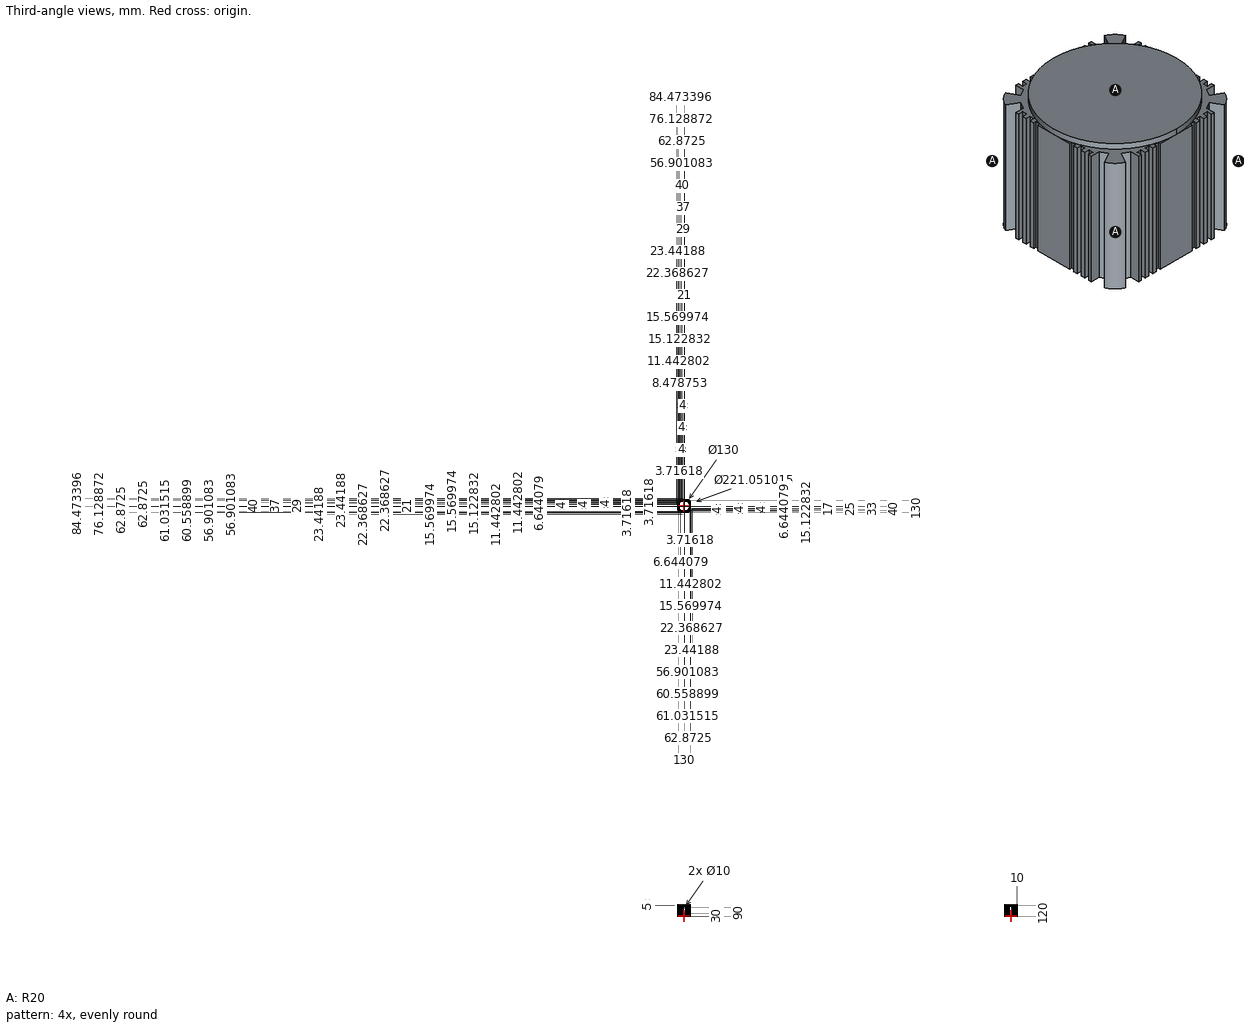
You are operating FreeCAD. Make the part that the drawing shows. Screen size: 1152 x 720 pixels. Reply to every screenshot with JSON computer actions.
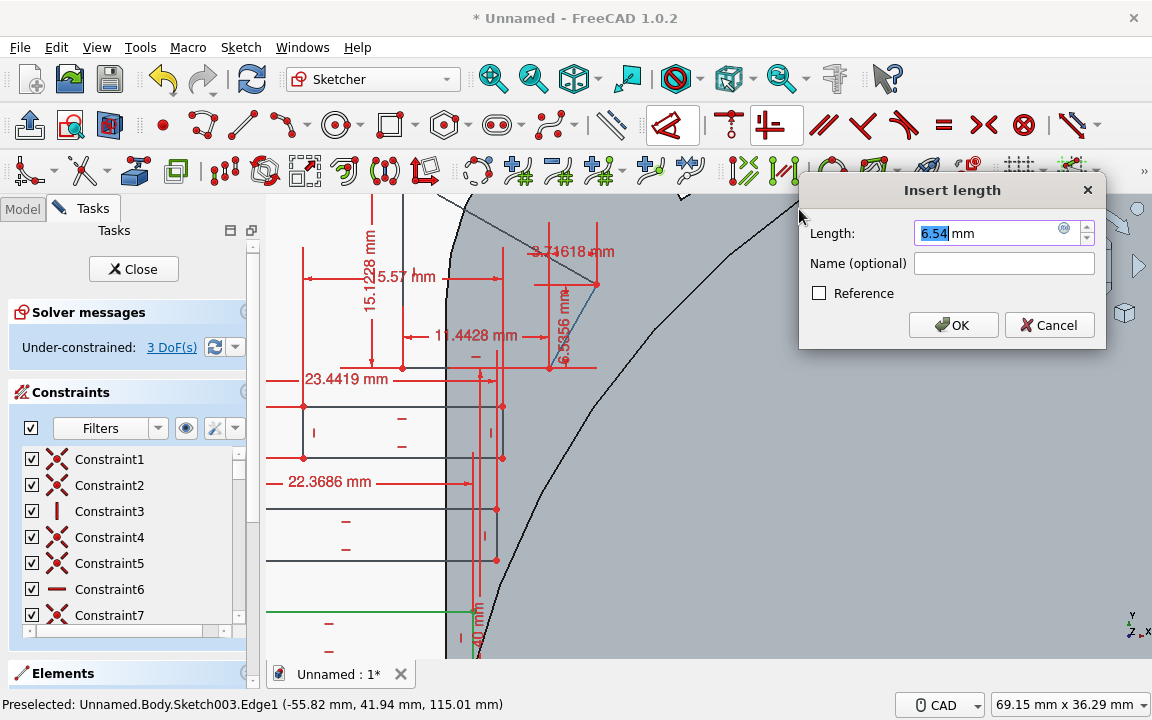
{"action": "type", "text": "6.644079"}
{"action": "key", "text": "Return"}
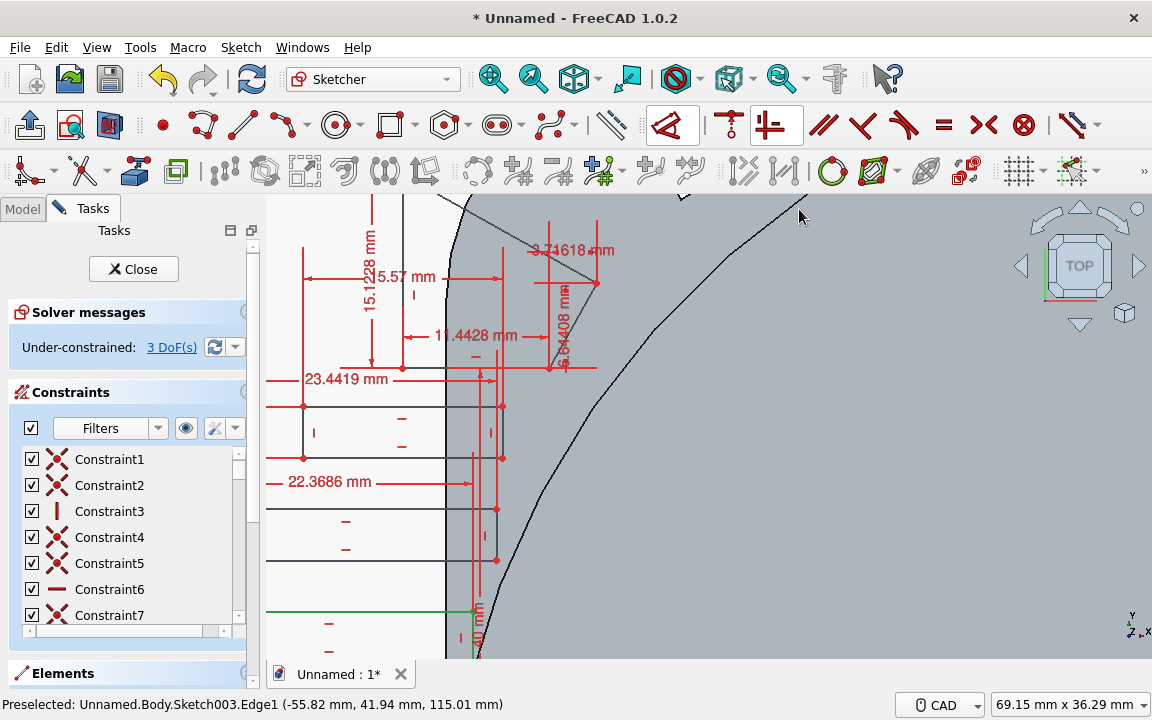
{"action": "left_click", "coordinate": [549, 368]}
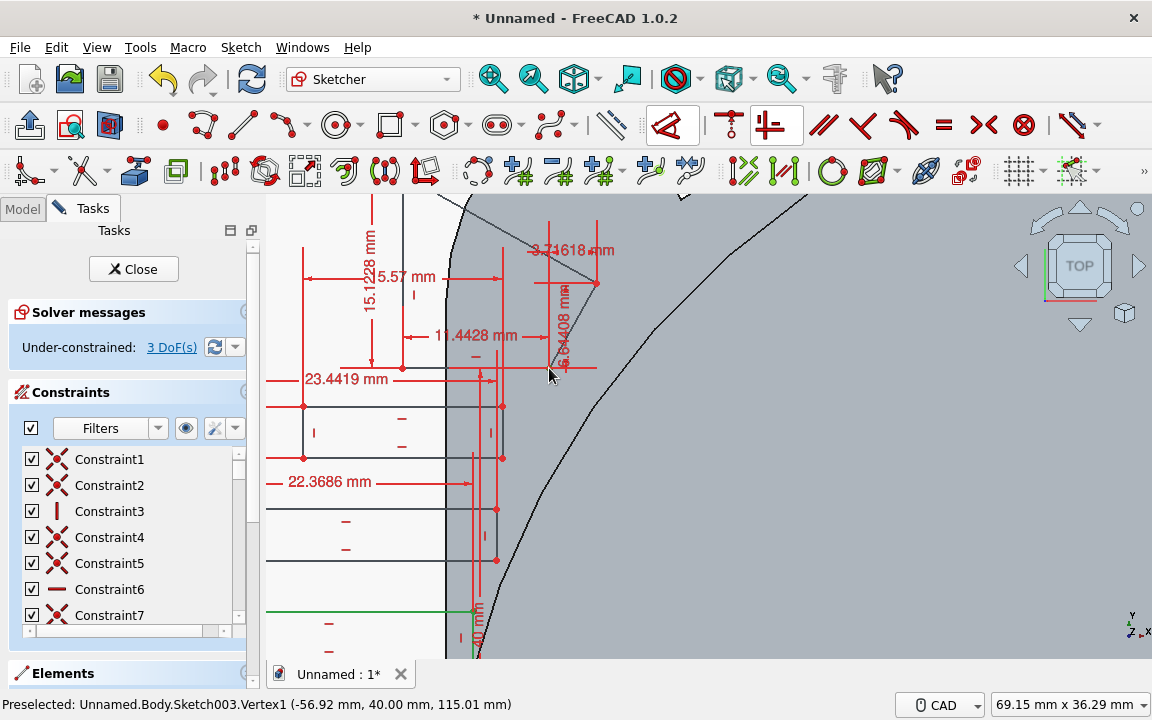
{"action": "left_click", "coordinate": [694, 126]}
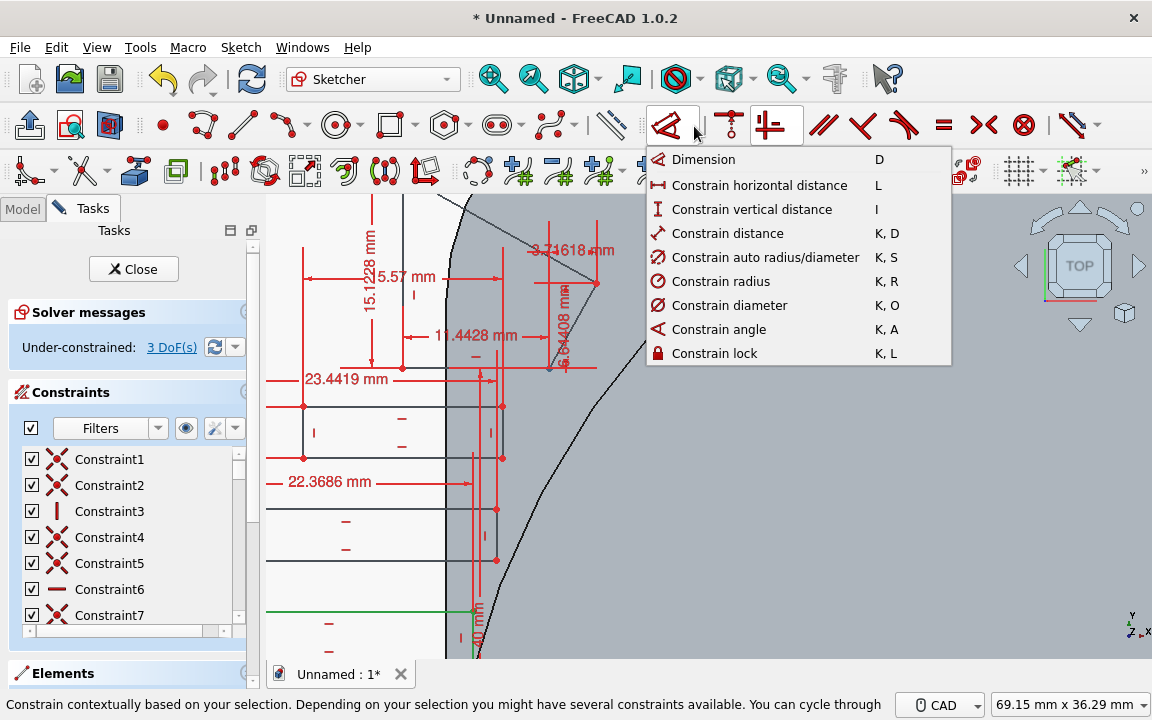
{"action": "left_click", "coordinate": [799, 185]}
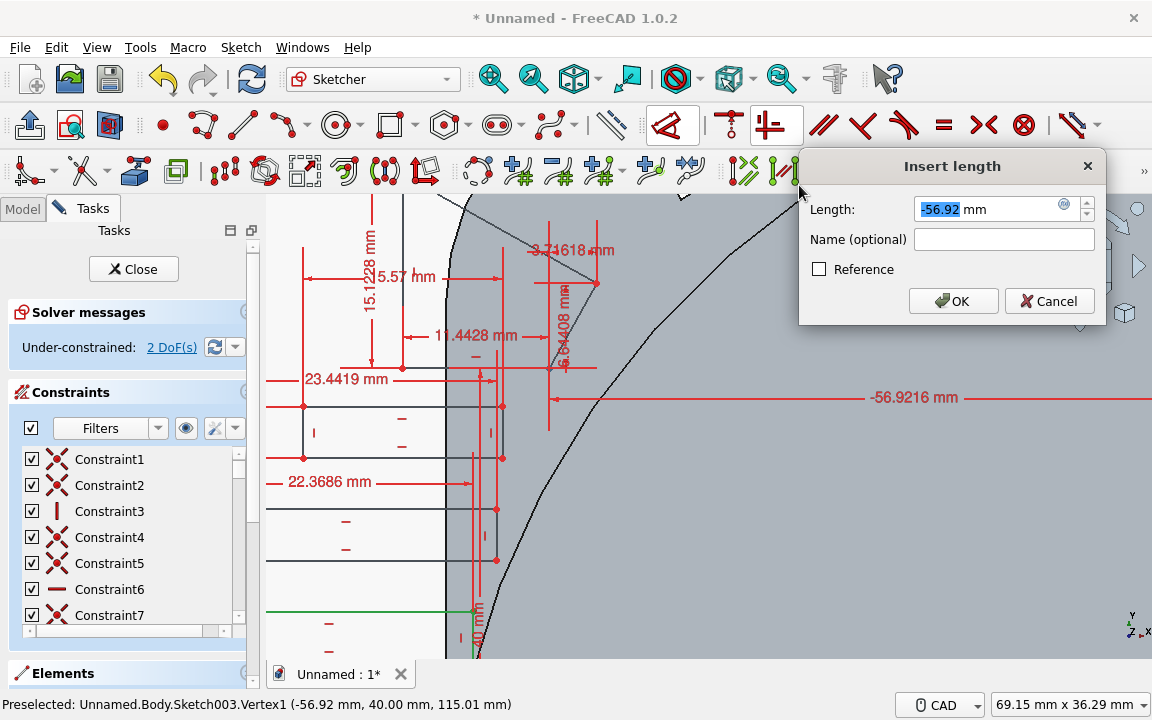
{"action": "type", "text": "-56.901083"}
{"action": "key", "text": "Return"}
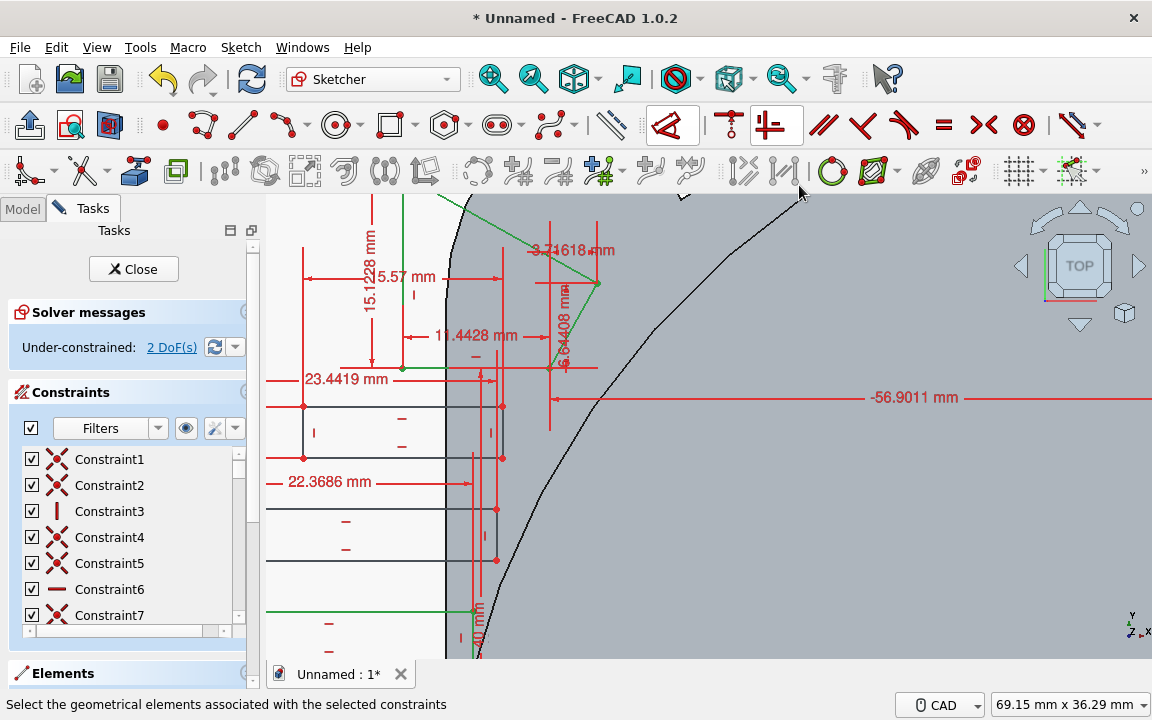
{"action": "left_click", "coordinate": [303, 407]}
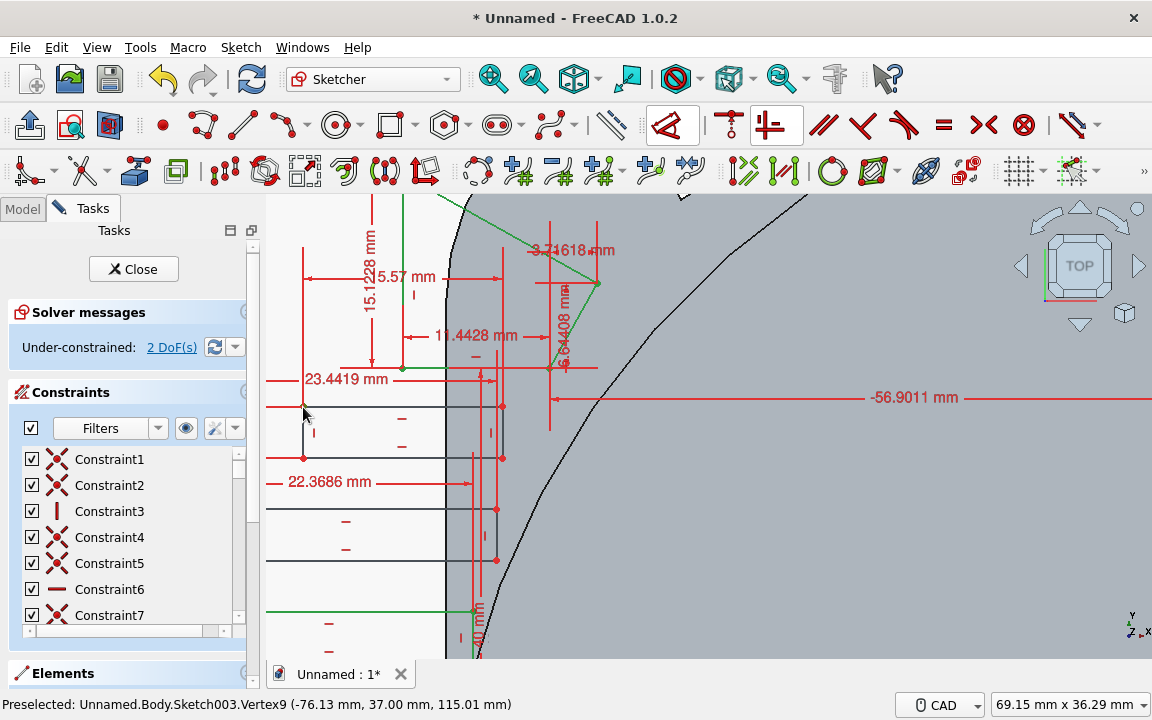
{"action": "left_click", "coordinate": [694, 126]}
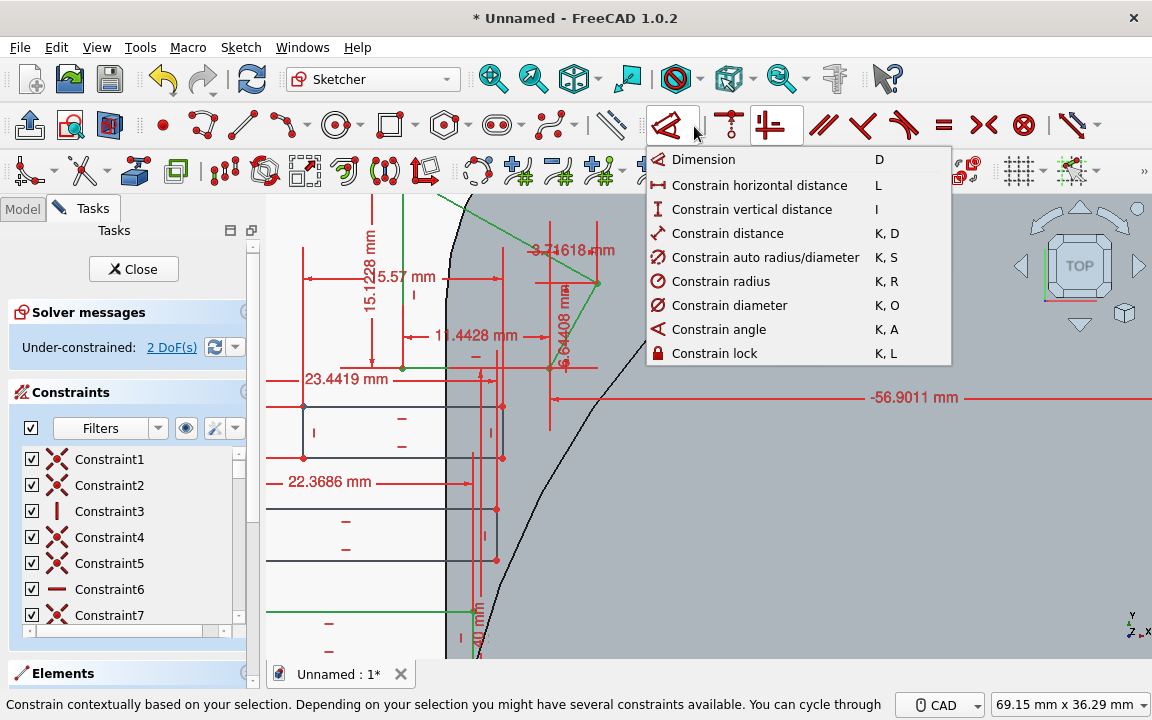
{"action": "left_click", "coordinate": [799, 185]}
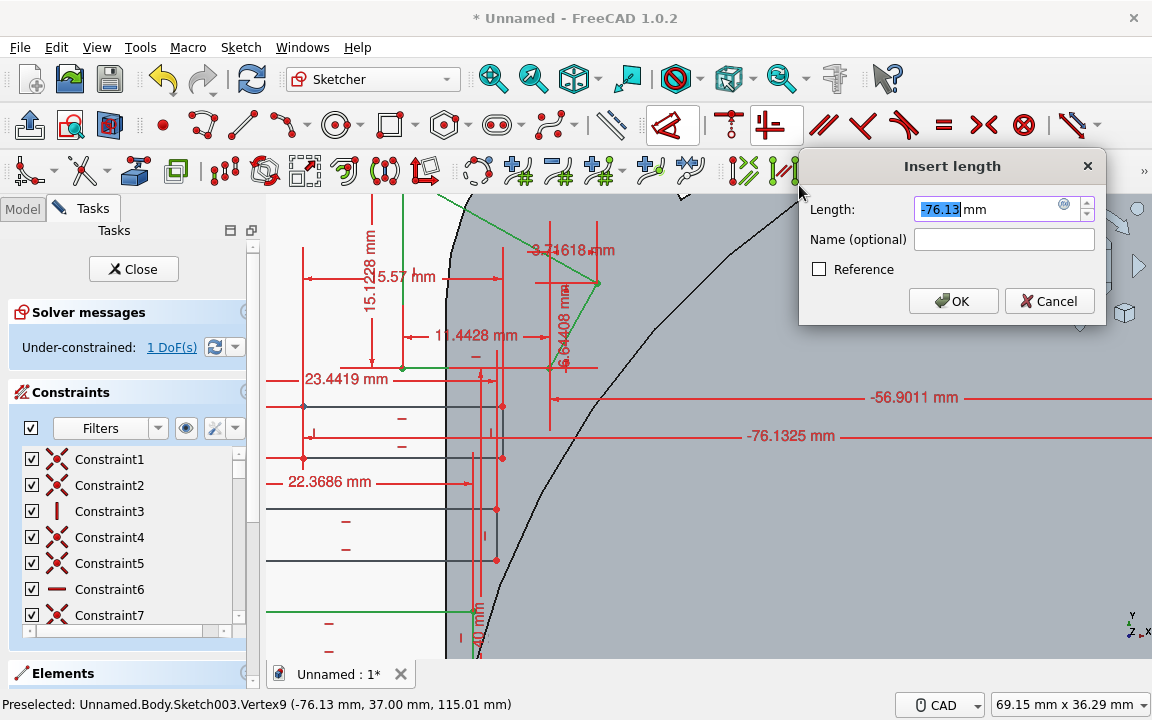
{"action": "type", "text": "-76.128872"}
{"action": "key", "text": "Return"}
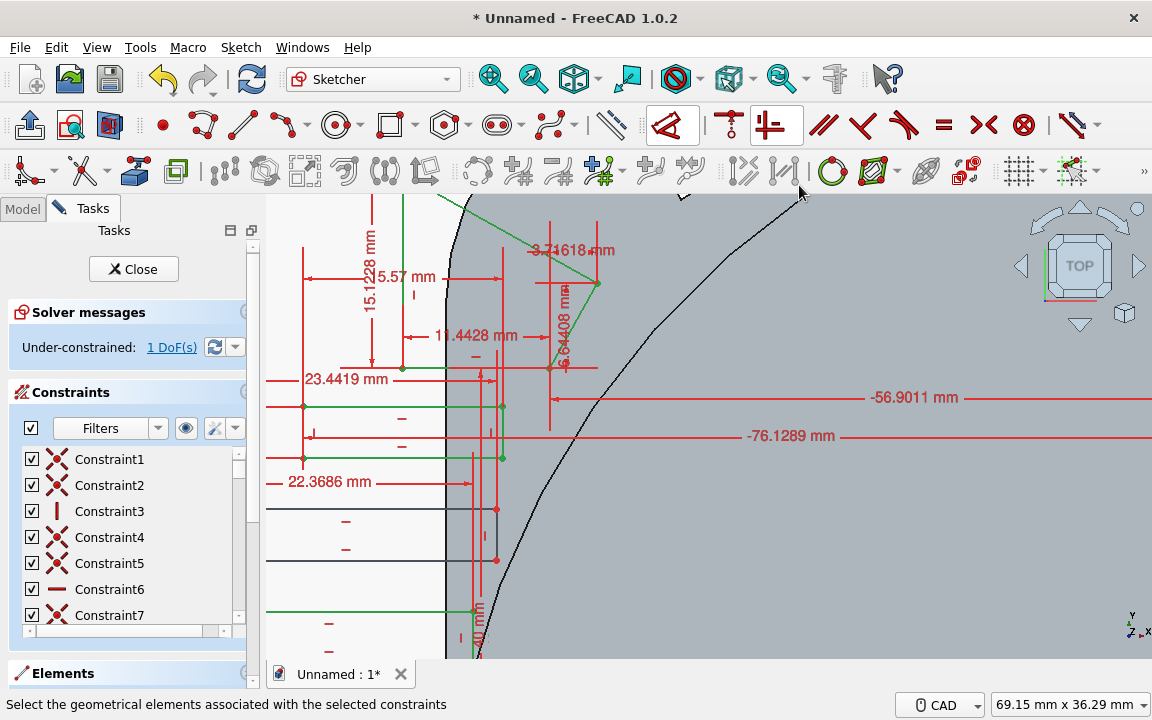
{"action": "scroll", "coordinate": [565, 344], "scroll_direction": "down", "scroll_amount": 4}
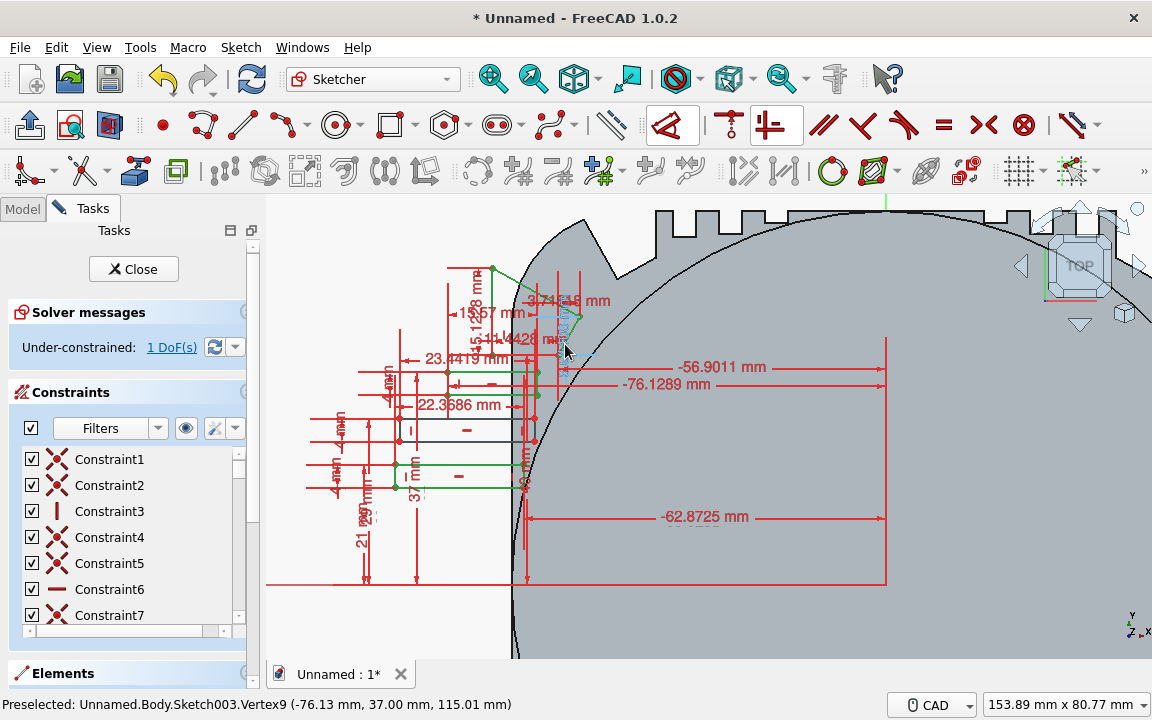
{"action": "left_click", "coordinate": [400, 419]}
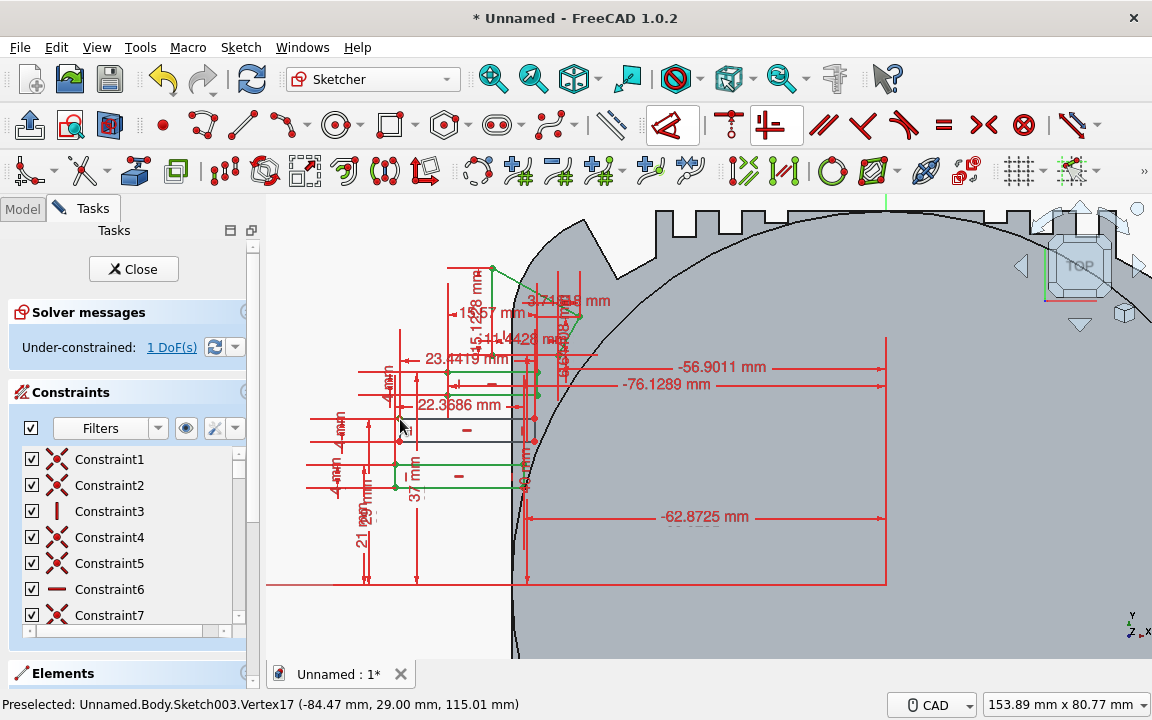
{"action": "key", "text": "l"}